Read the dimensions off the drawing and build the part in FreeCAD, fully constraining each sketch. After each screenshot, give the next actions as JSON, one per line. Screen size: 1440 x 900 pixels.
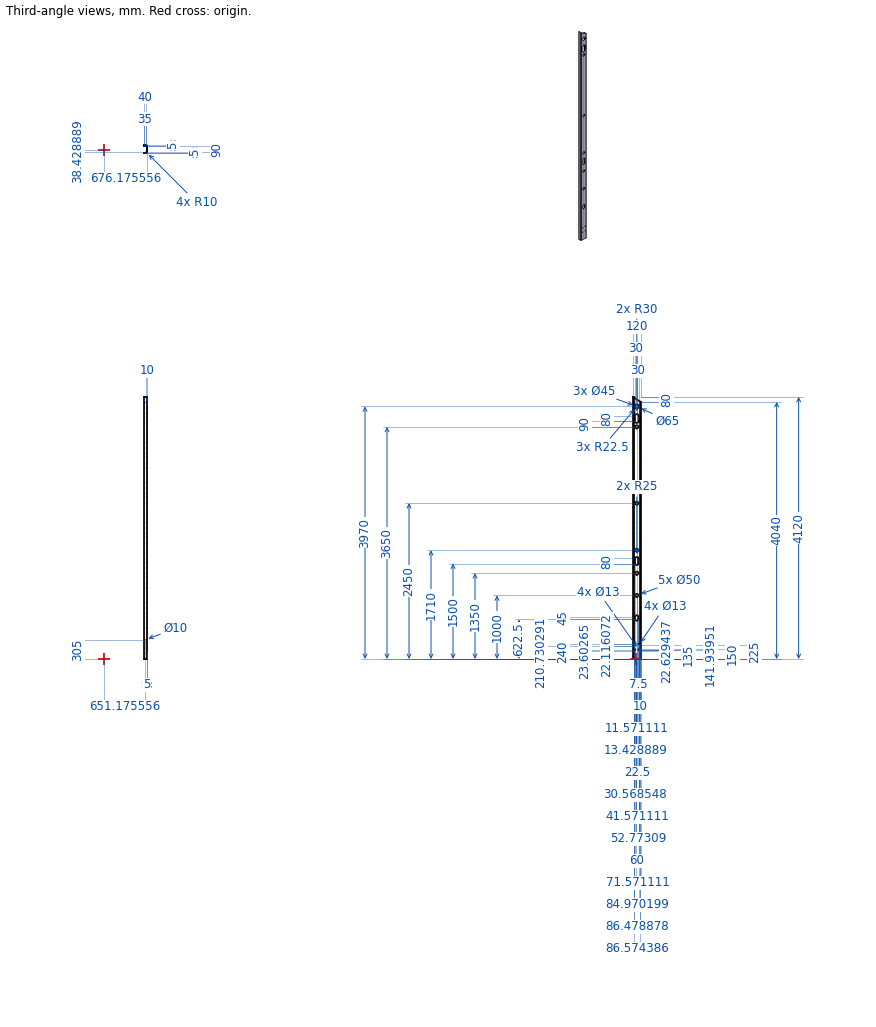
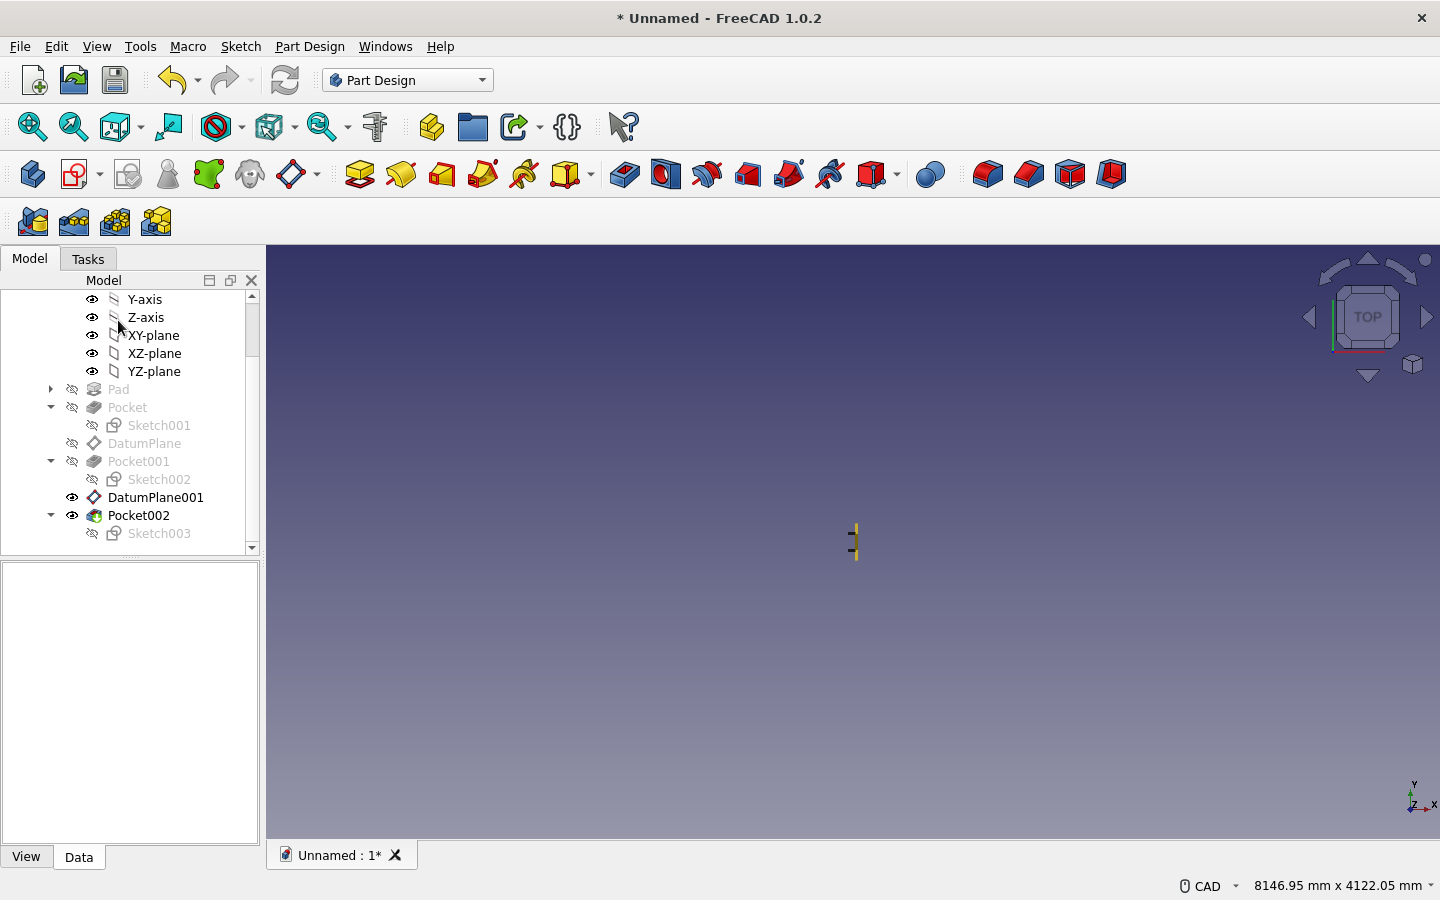
{"action": "left_click", "coordinate": [117, 497]}
{"action": "key", "text": "space"}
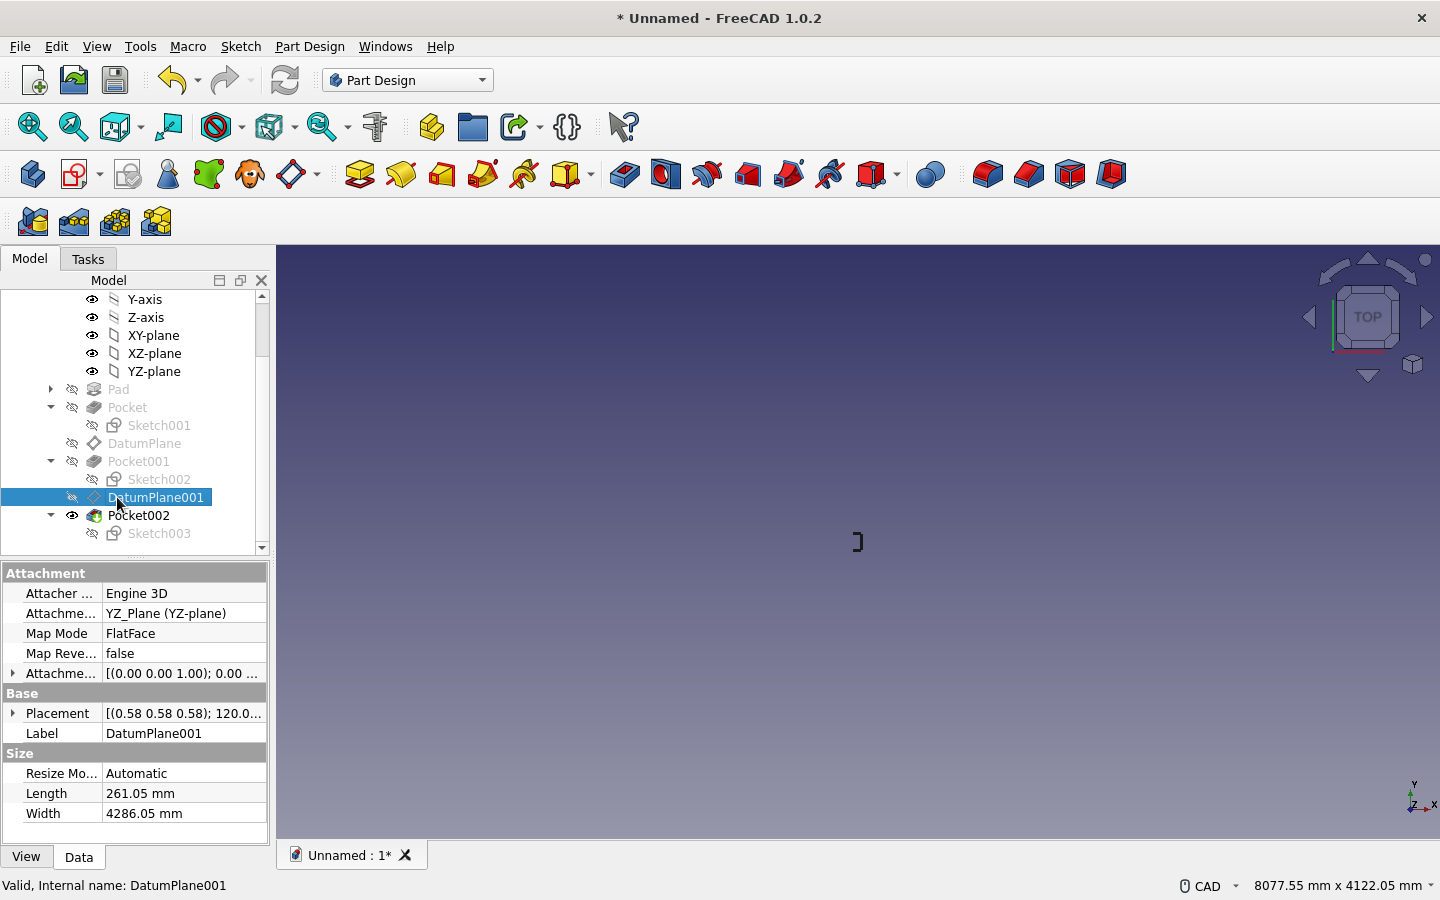
{"action": "key", "text": "v f"}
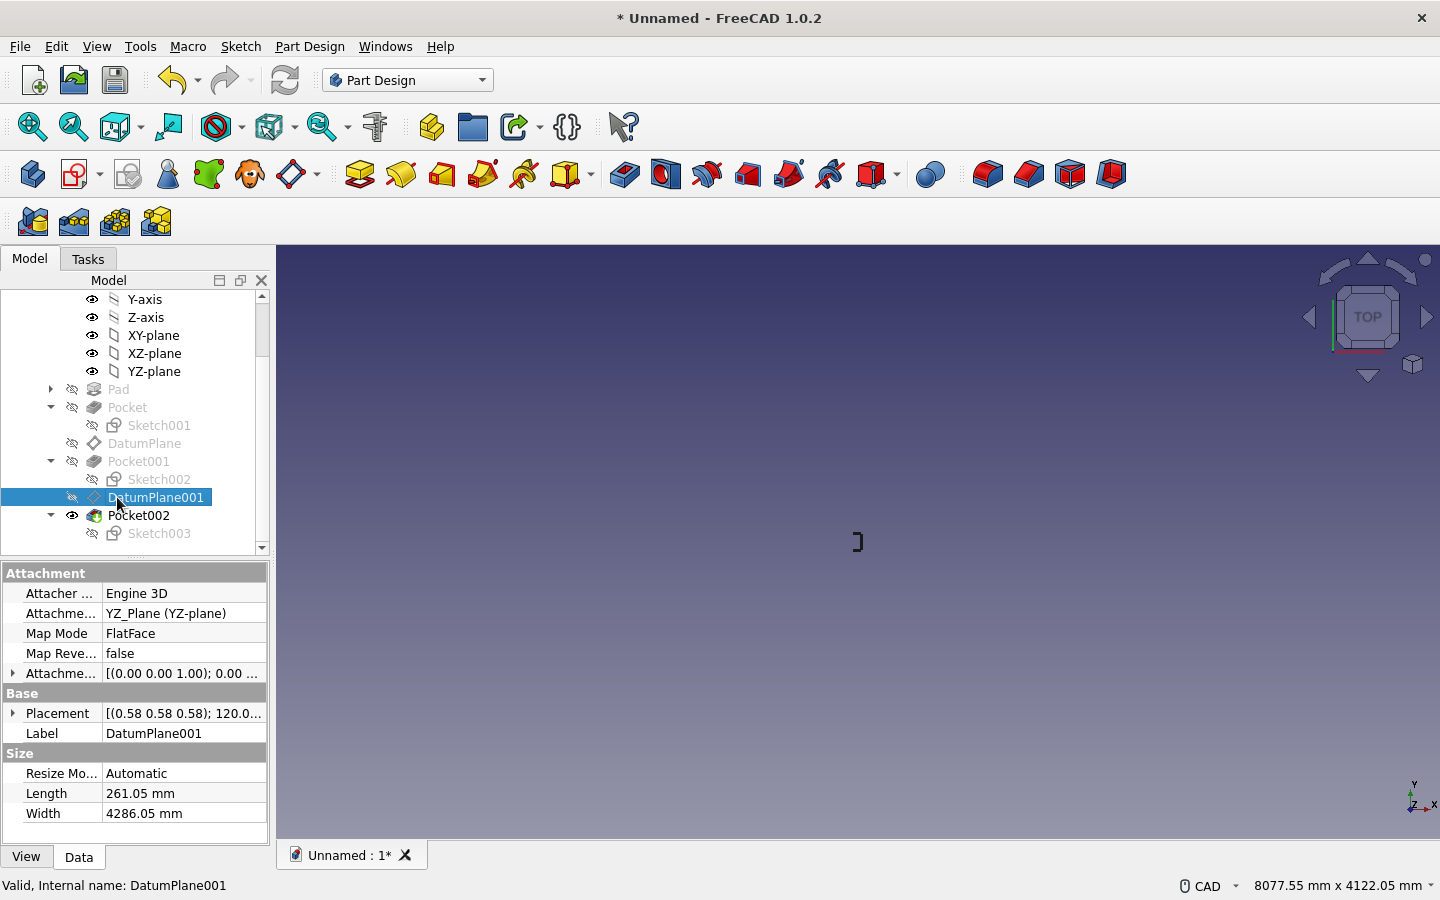
{"action": "key", "text": "0"}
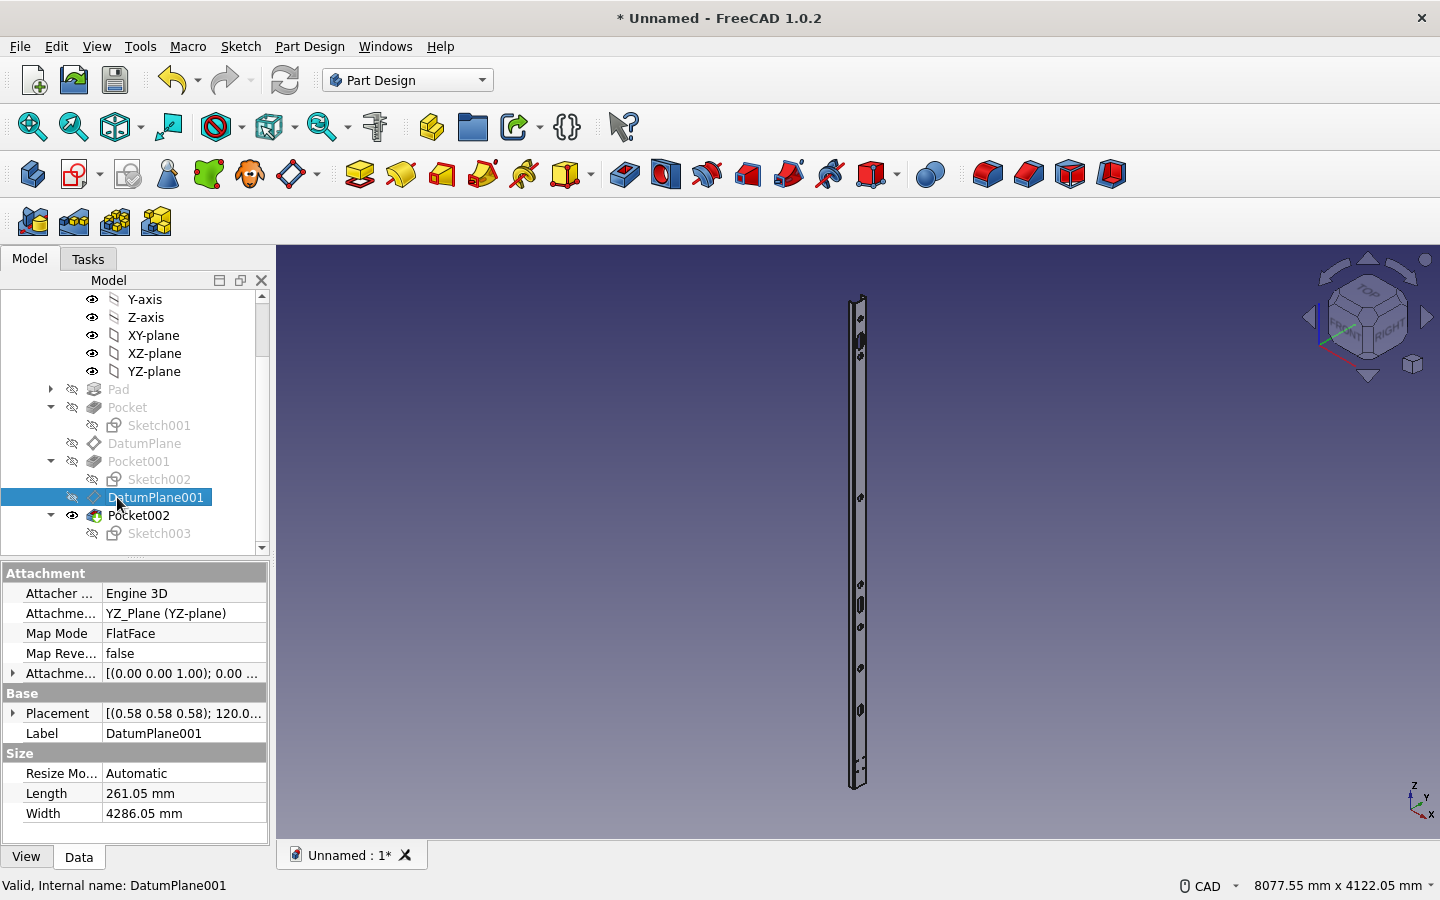
{"action": "key", "text": "3"}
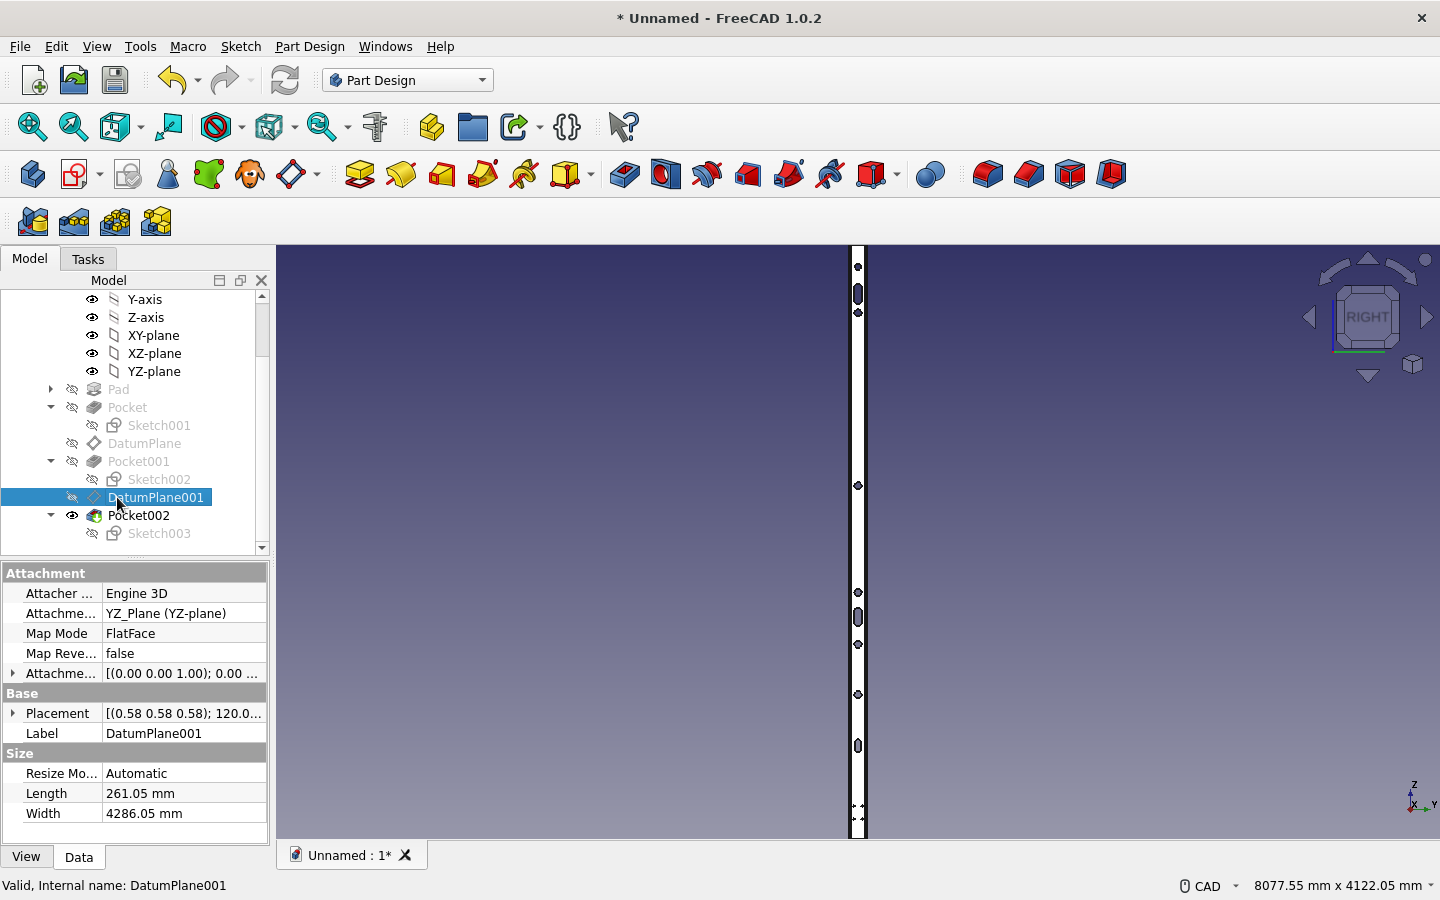
{"action": "key", "text": "v f"}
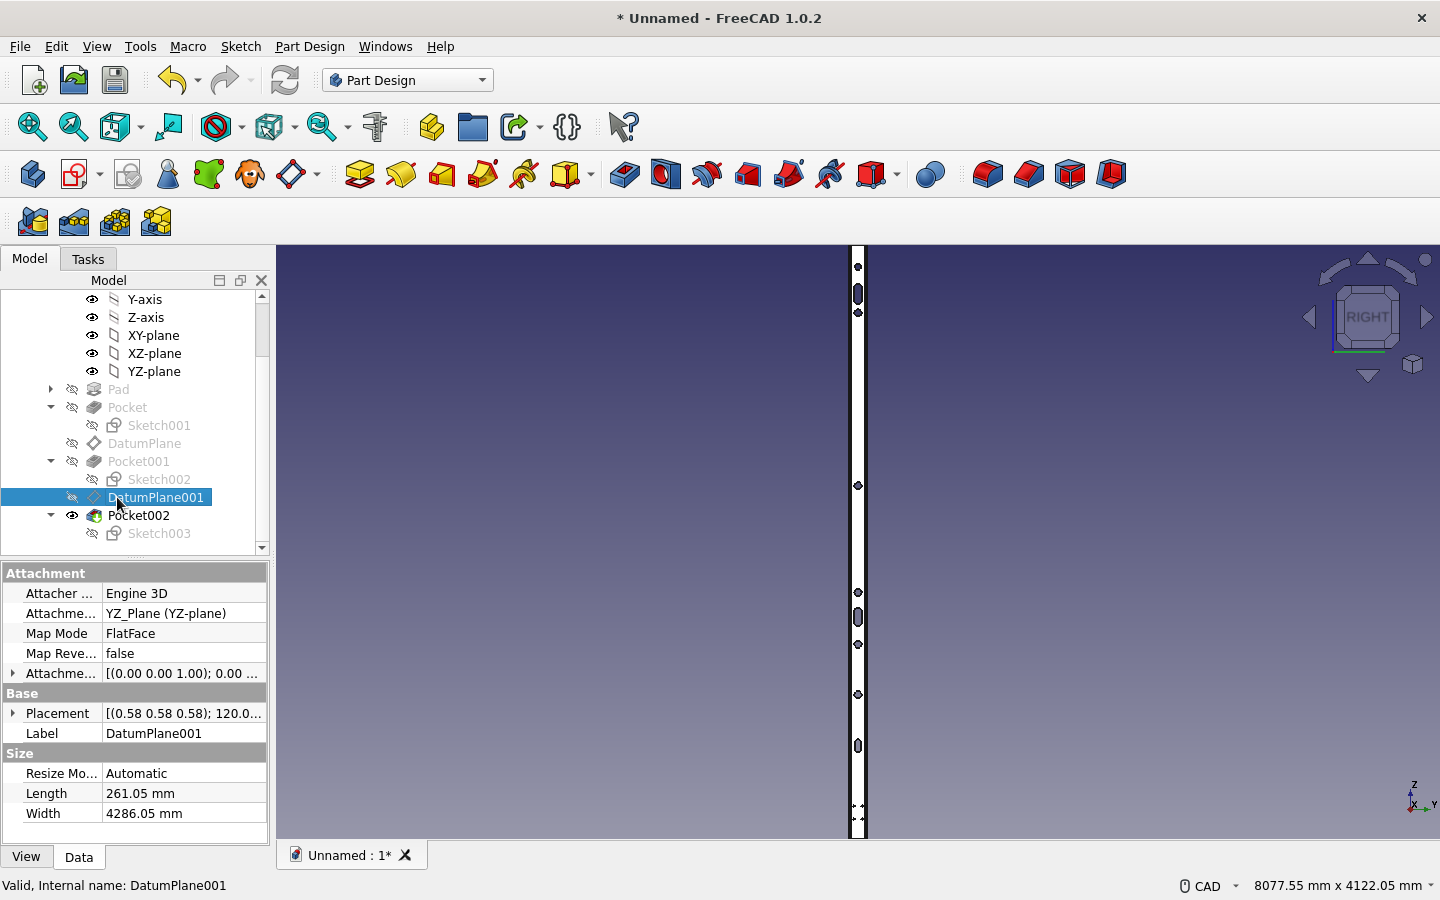
{"action": "key", "text": "2"}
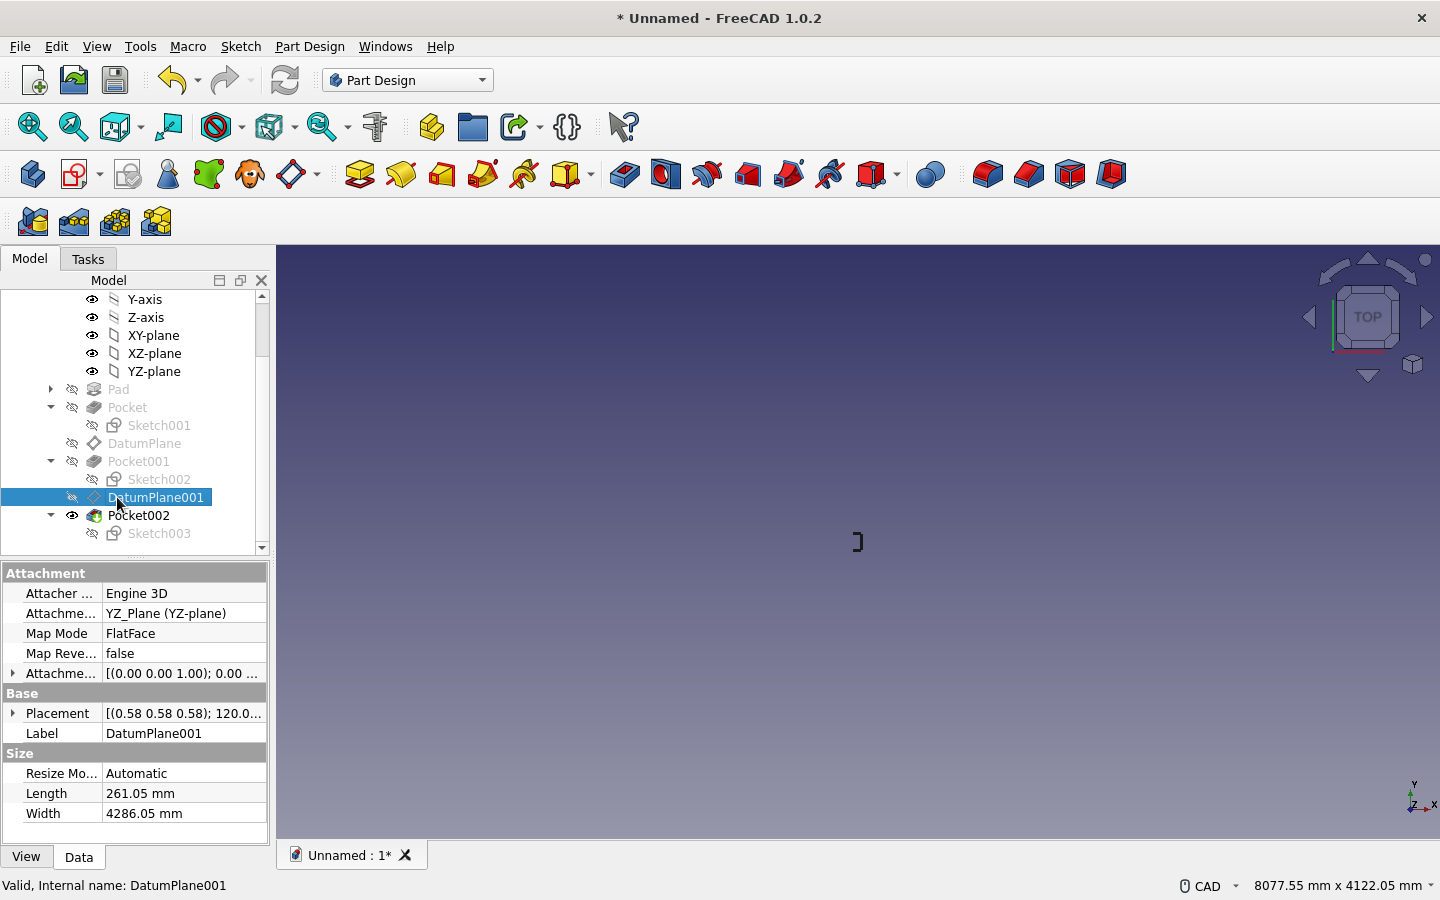
{"action": "key", "text": "v f"}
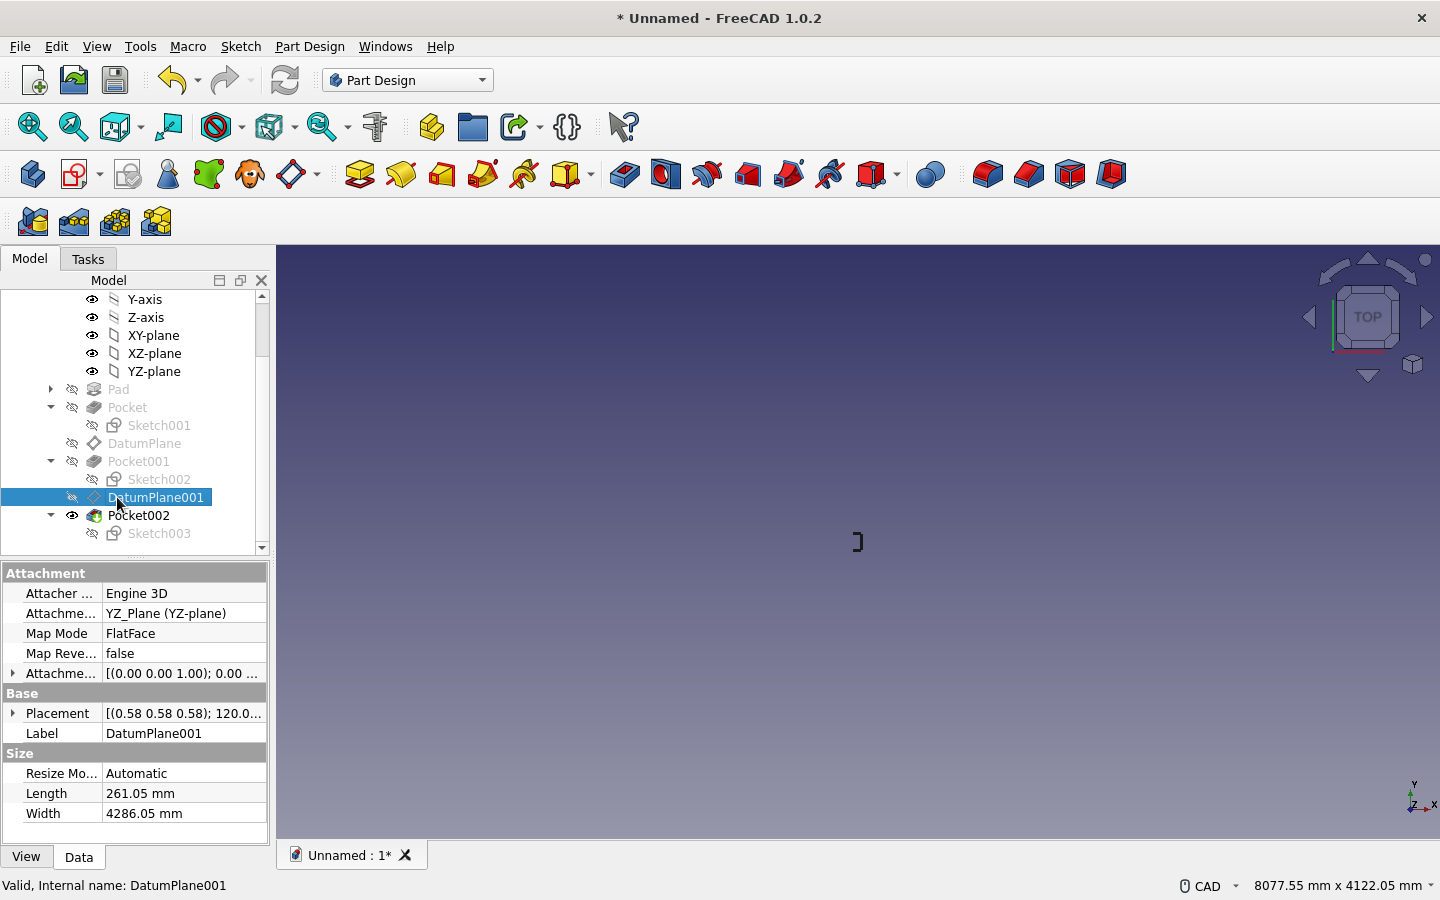
{"action": "scroll", "coordinate": [161, 421], "scroll_direction": "down", "scroll_amount": 3}